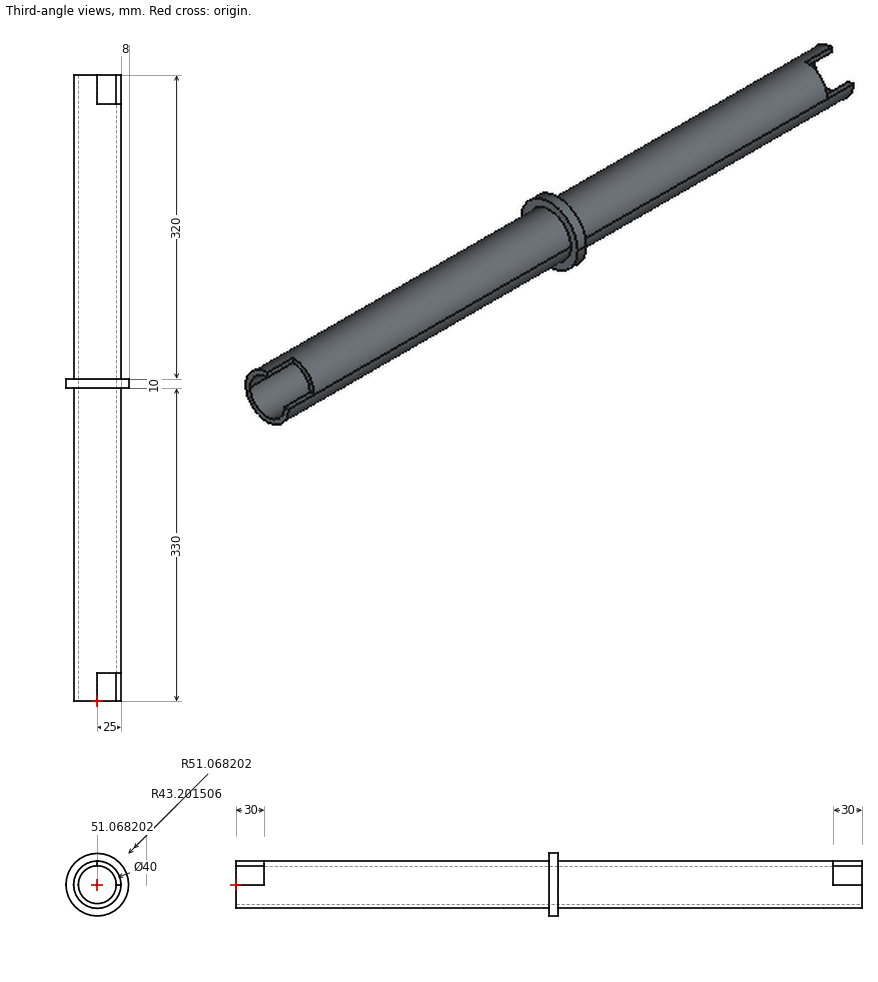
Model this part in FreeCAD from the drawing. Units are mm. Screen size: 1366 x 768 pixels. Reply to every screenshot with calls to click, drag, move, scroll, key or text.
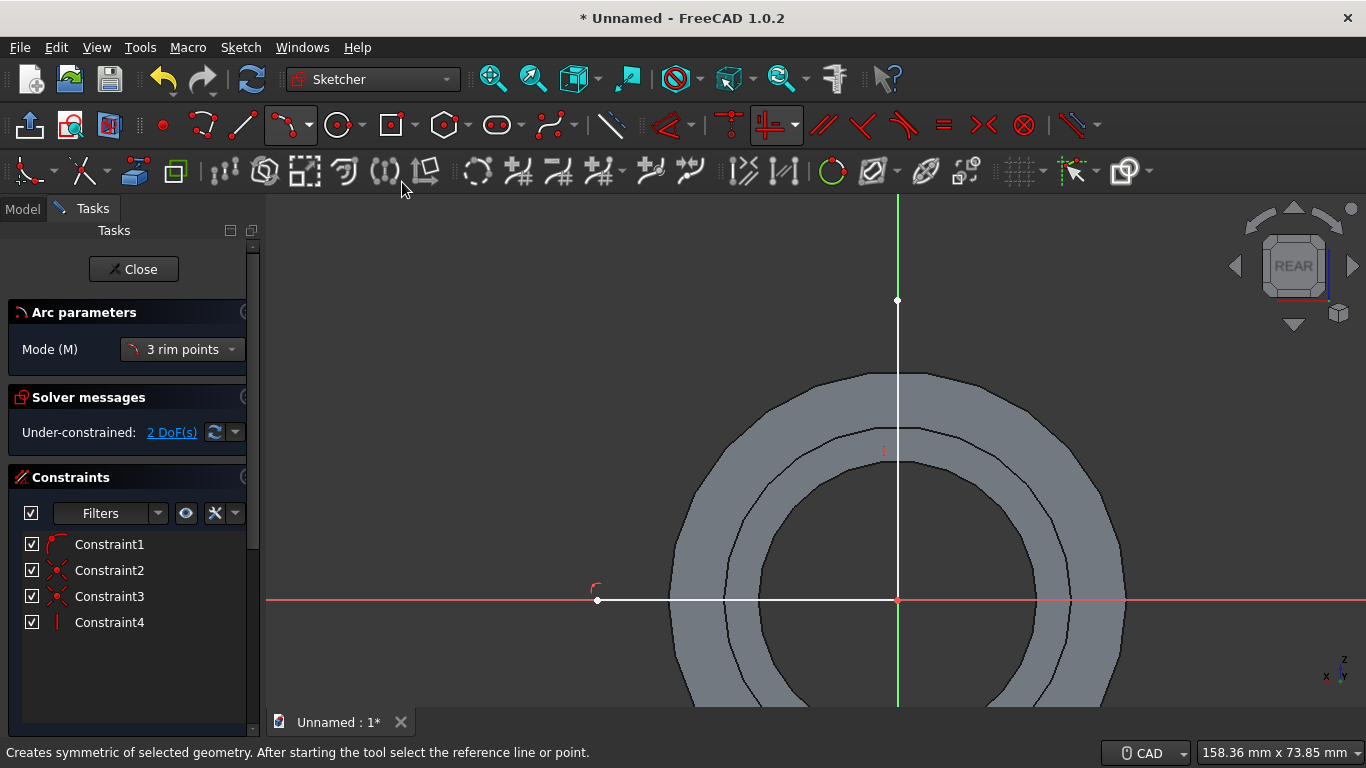
click(898, 301)
click(597, 600)
click(685, 388)
key(Escape)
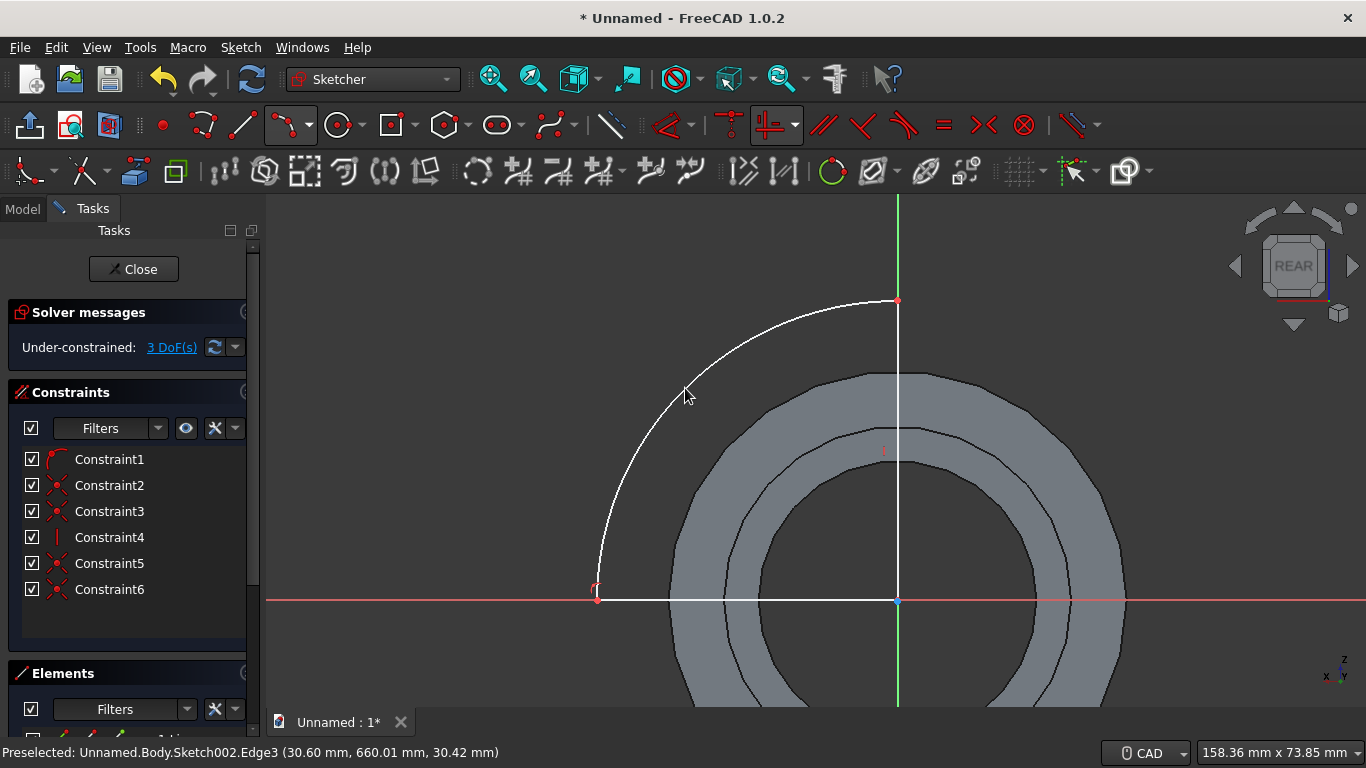
scroll(897, 601, up, 22)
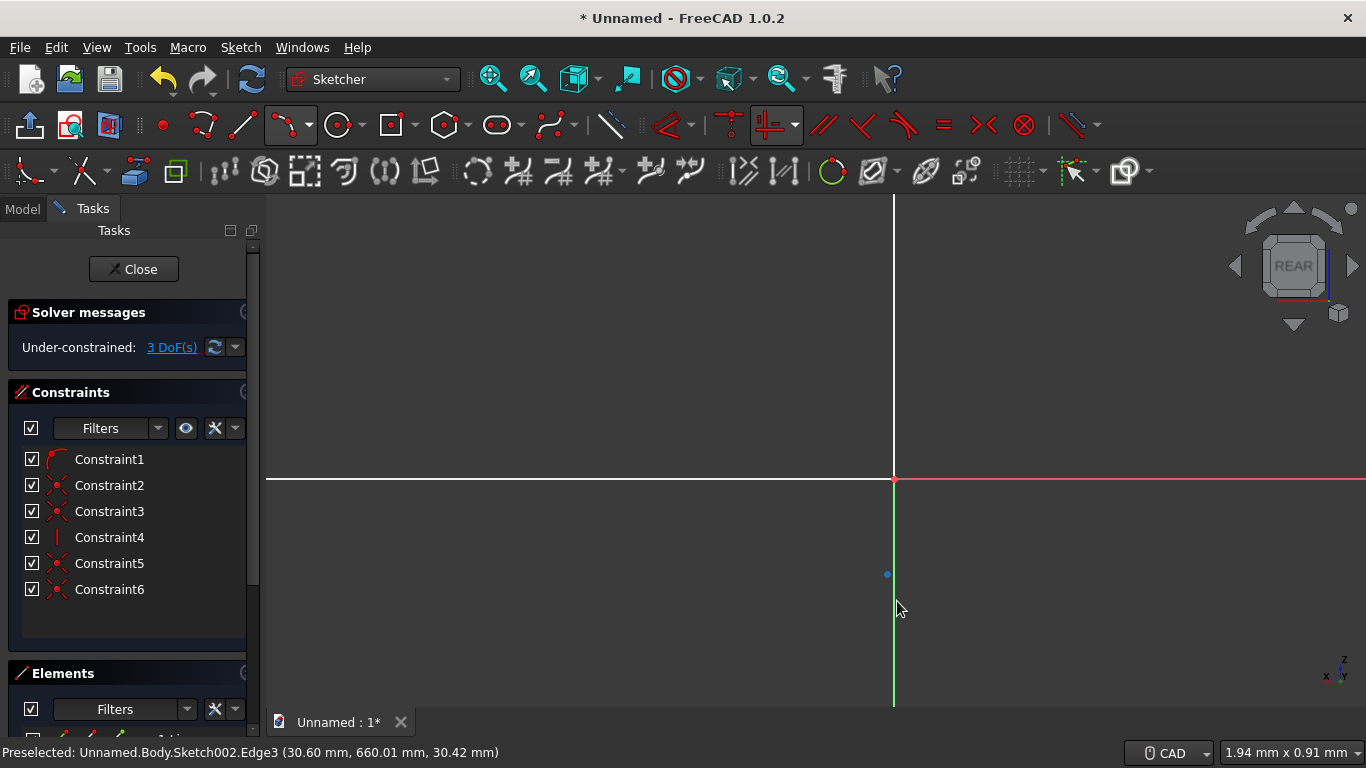
drag(878, 469, 904, 584)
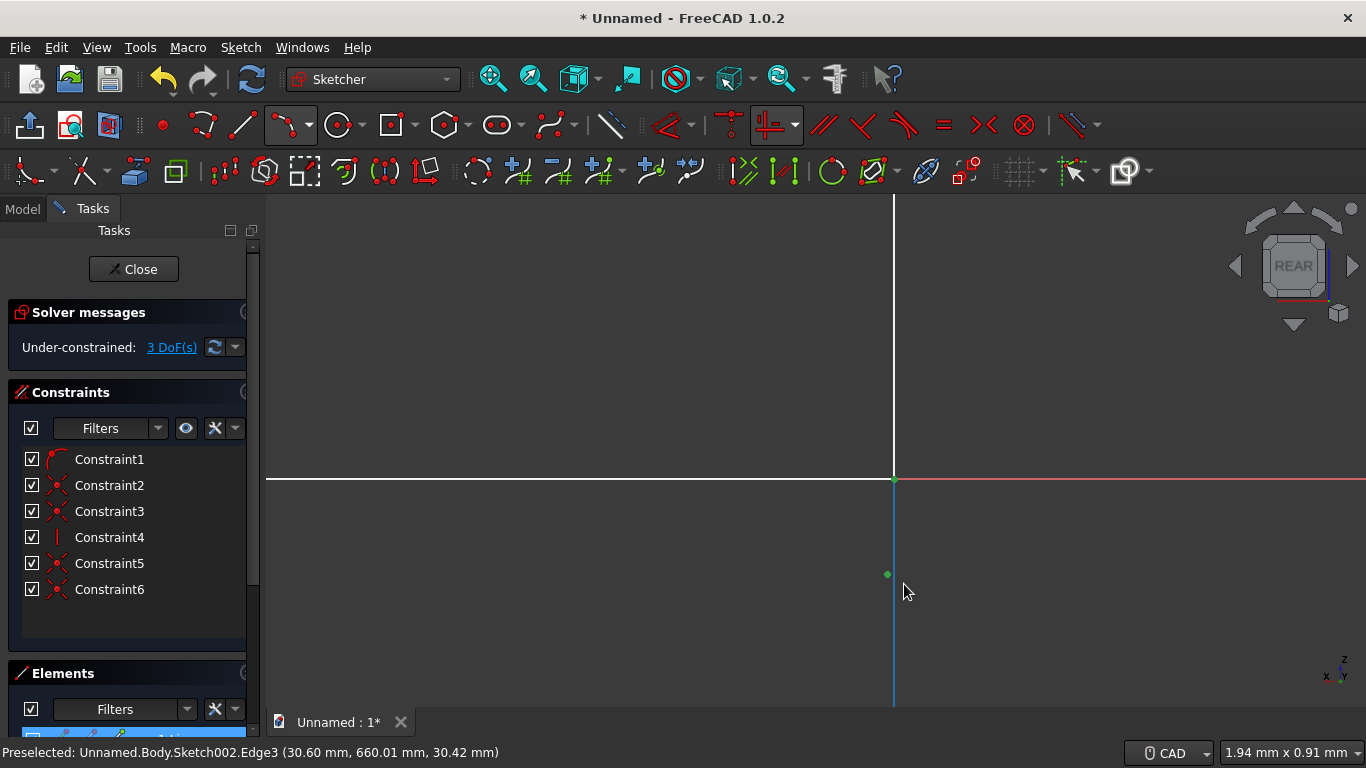
click(730, 126)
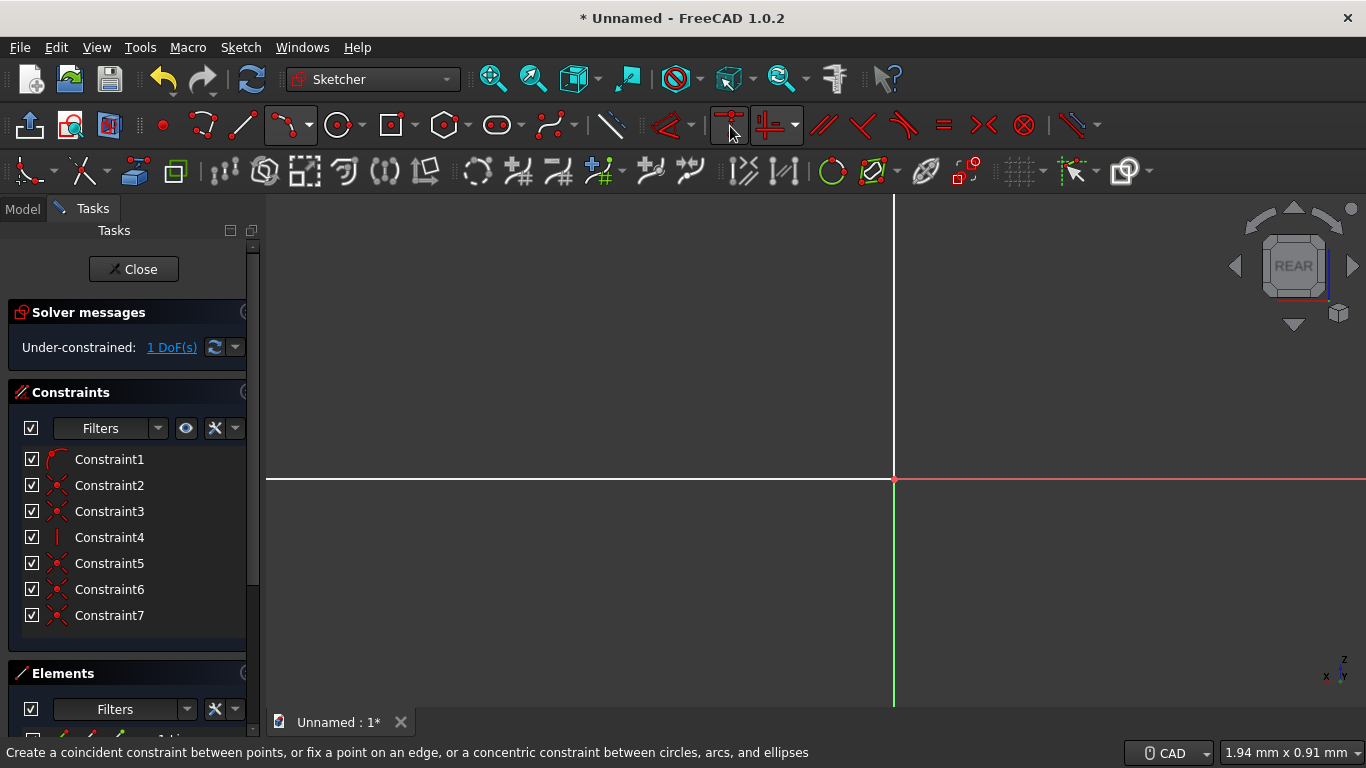
click(666, 126)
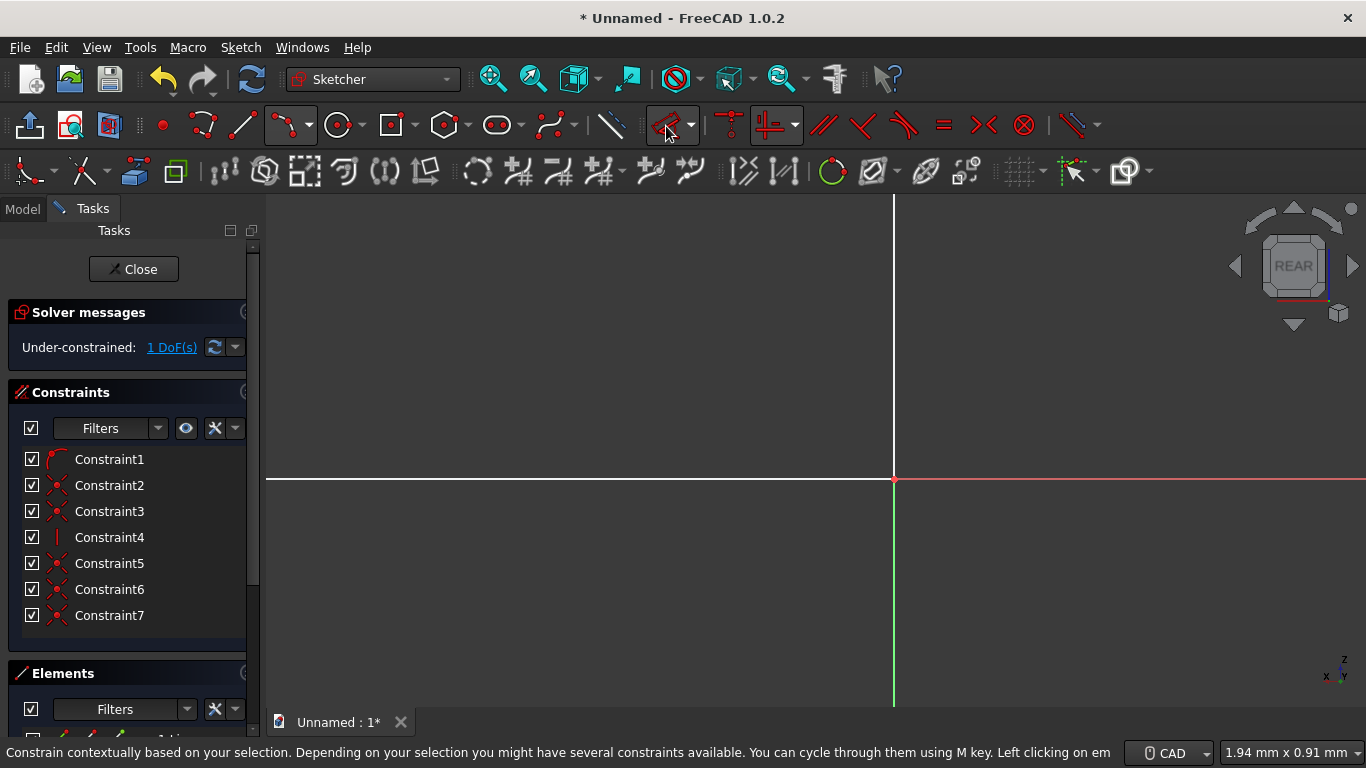
scroll(748, 450, down, 15)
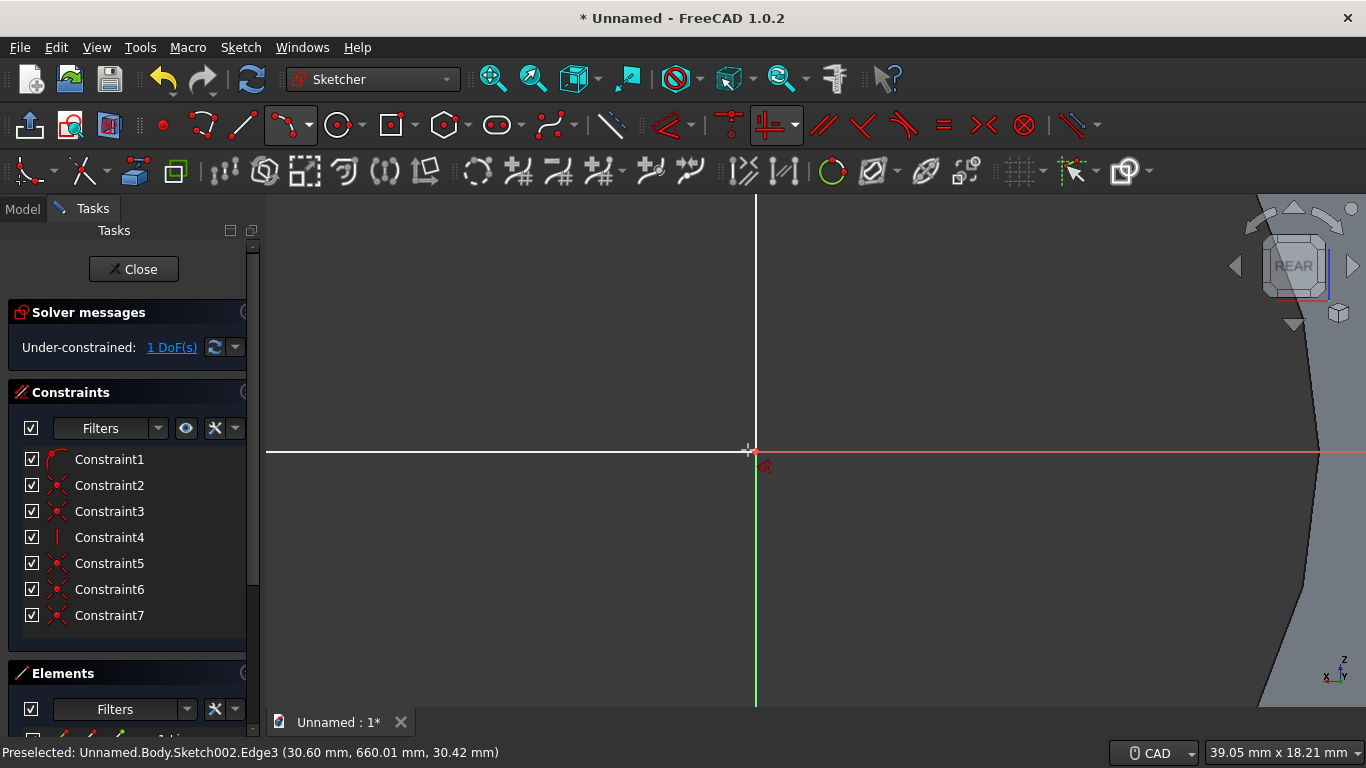
scroll(944, 649, down, 7)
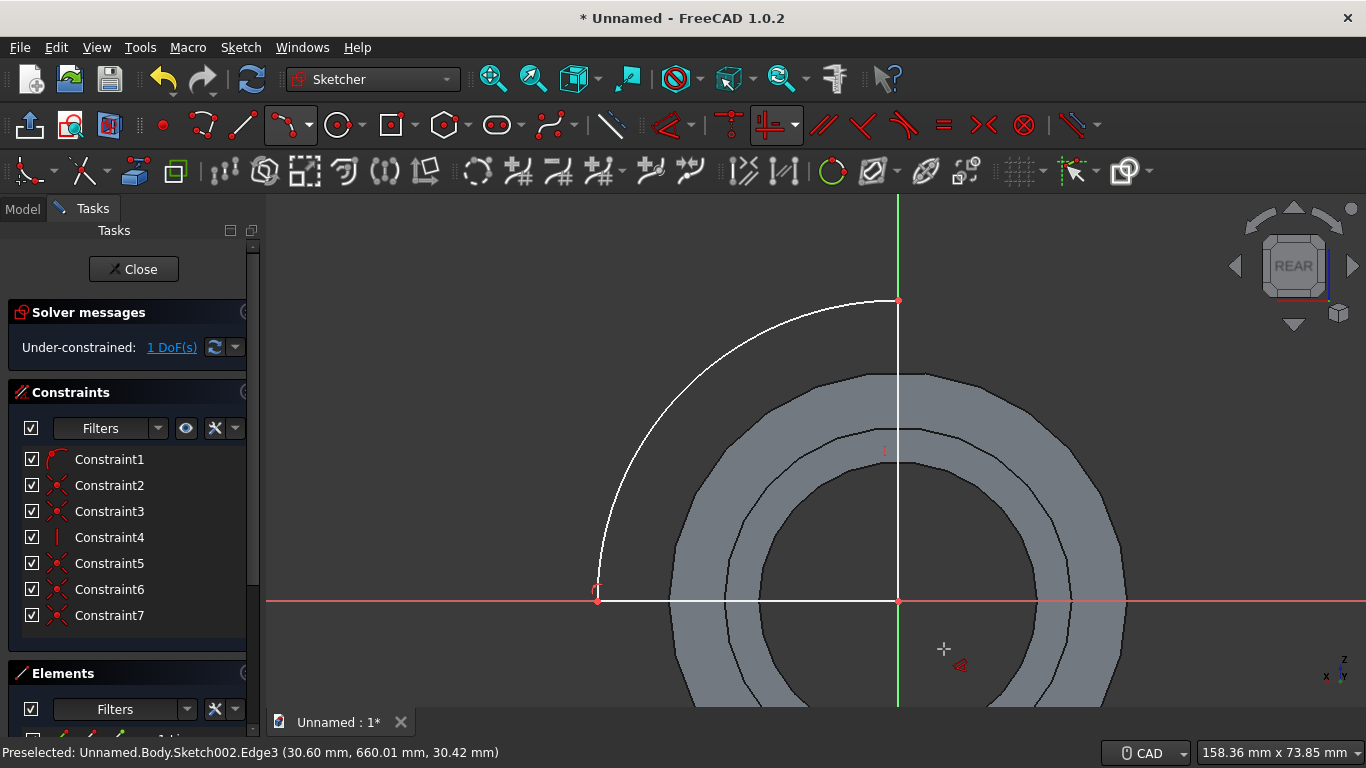
click(762, 333)
click(748, 304)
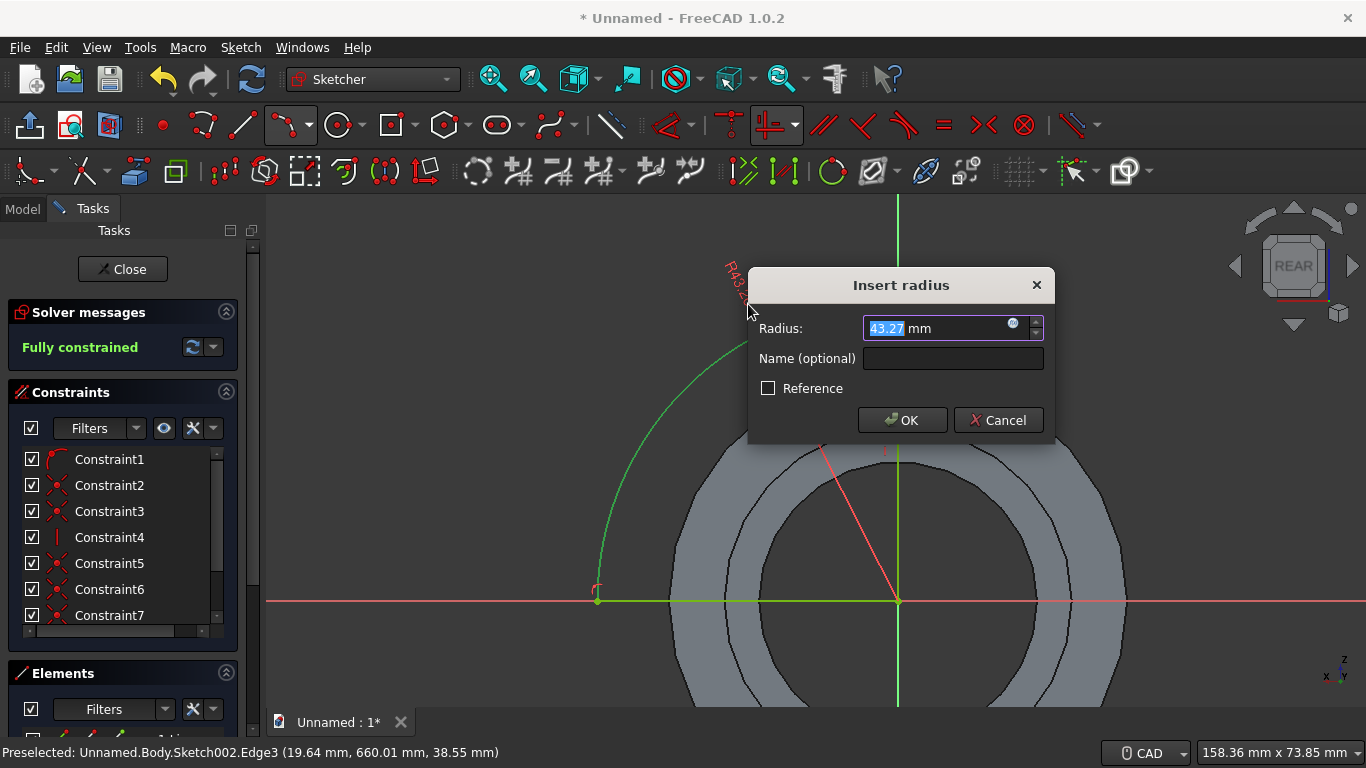
text(43.201506)
key(Return)
key(Escape)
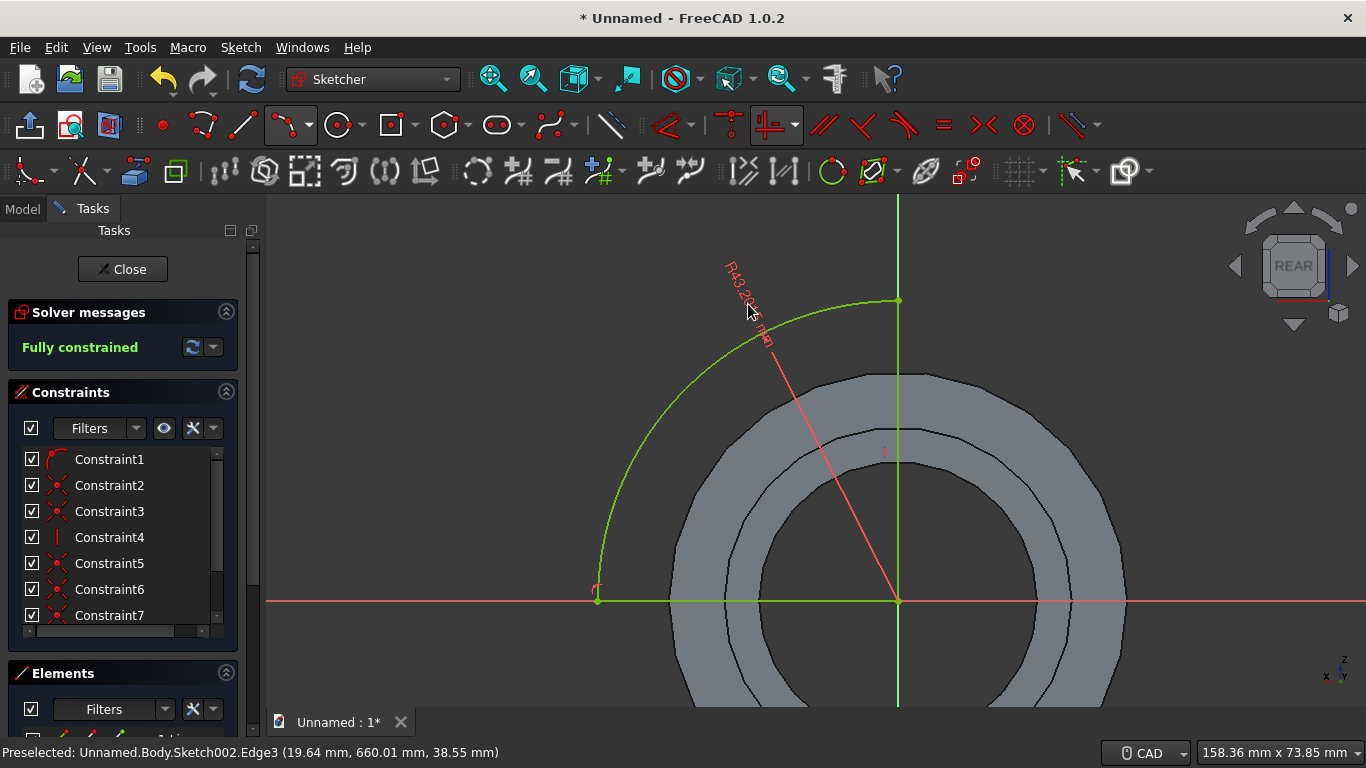
click(123, 269)